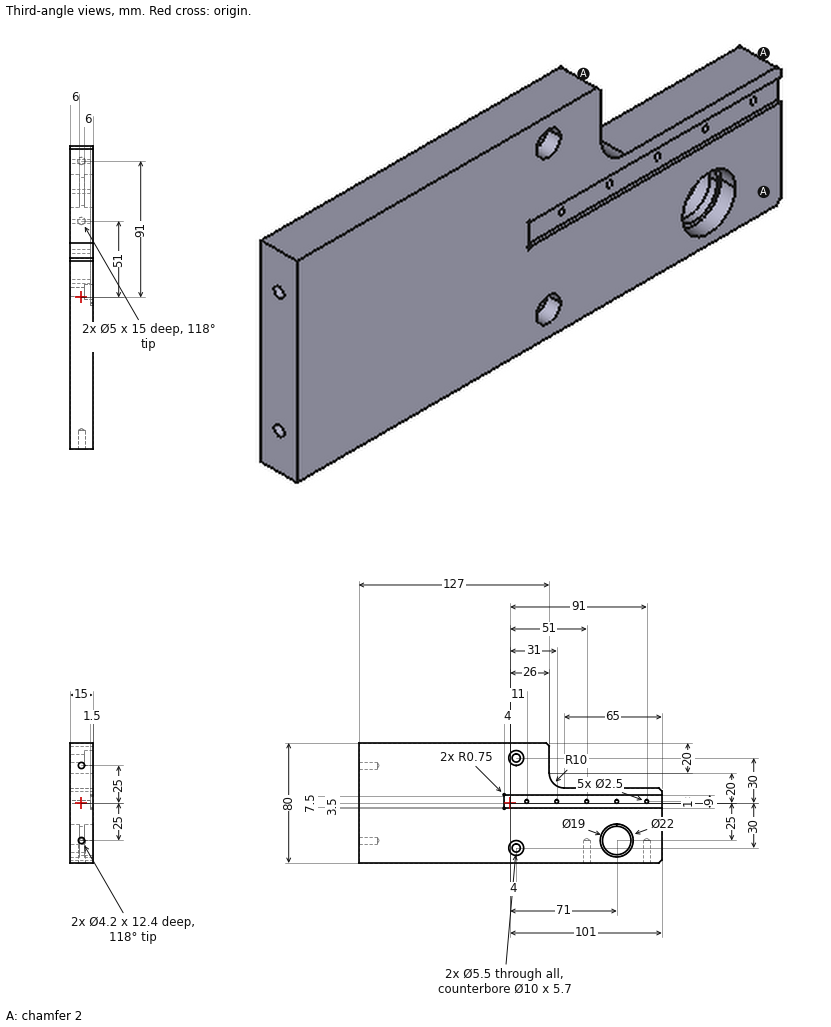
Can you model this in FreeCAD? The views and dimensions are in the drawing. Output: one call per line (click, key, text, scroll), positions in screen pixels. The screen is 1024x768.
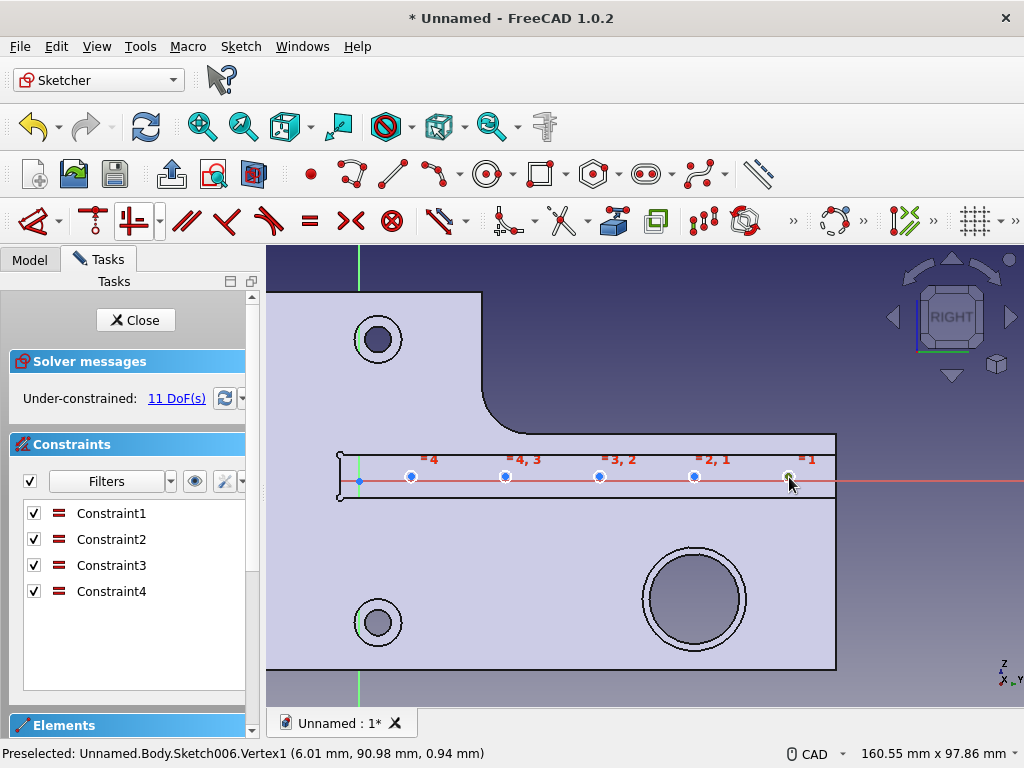
click(694, 477)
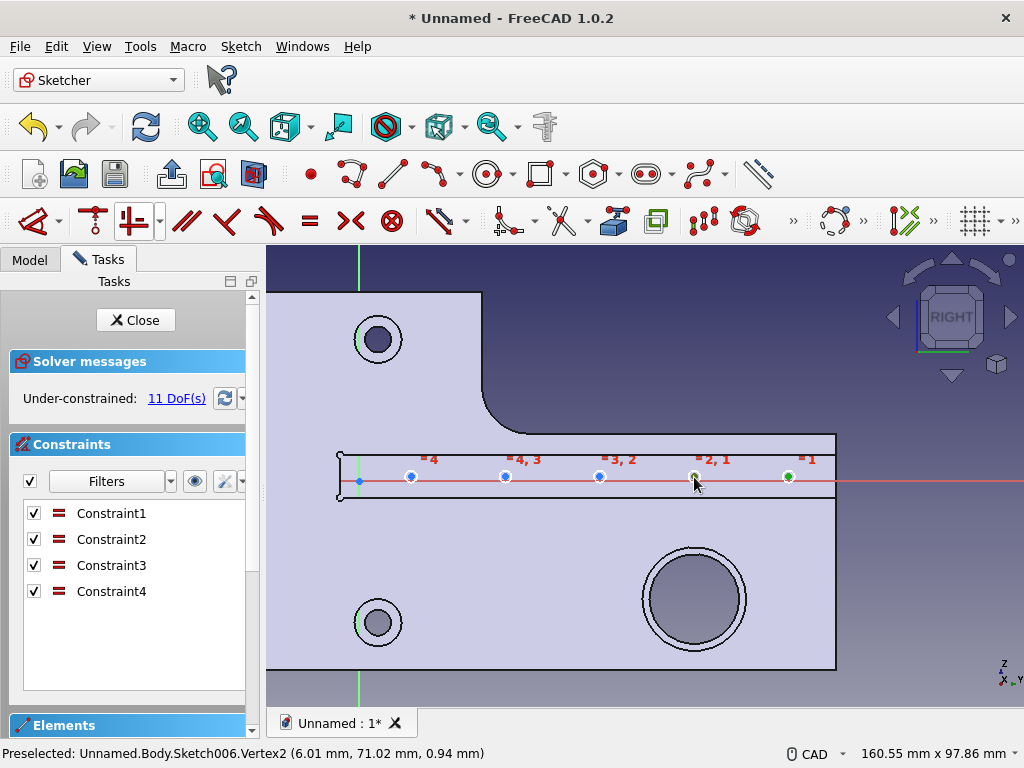
key(h)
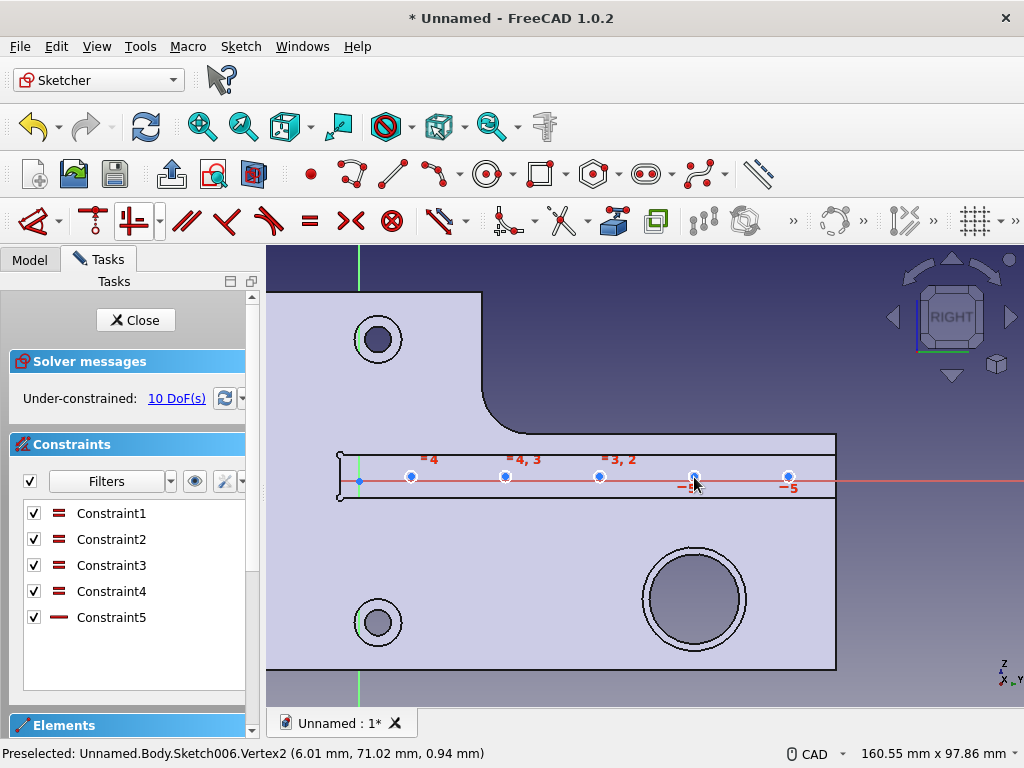
click(694, 477)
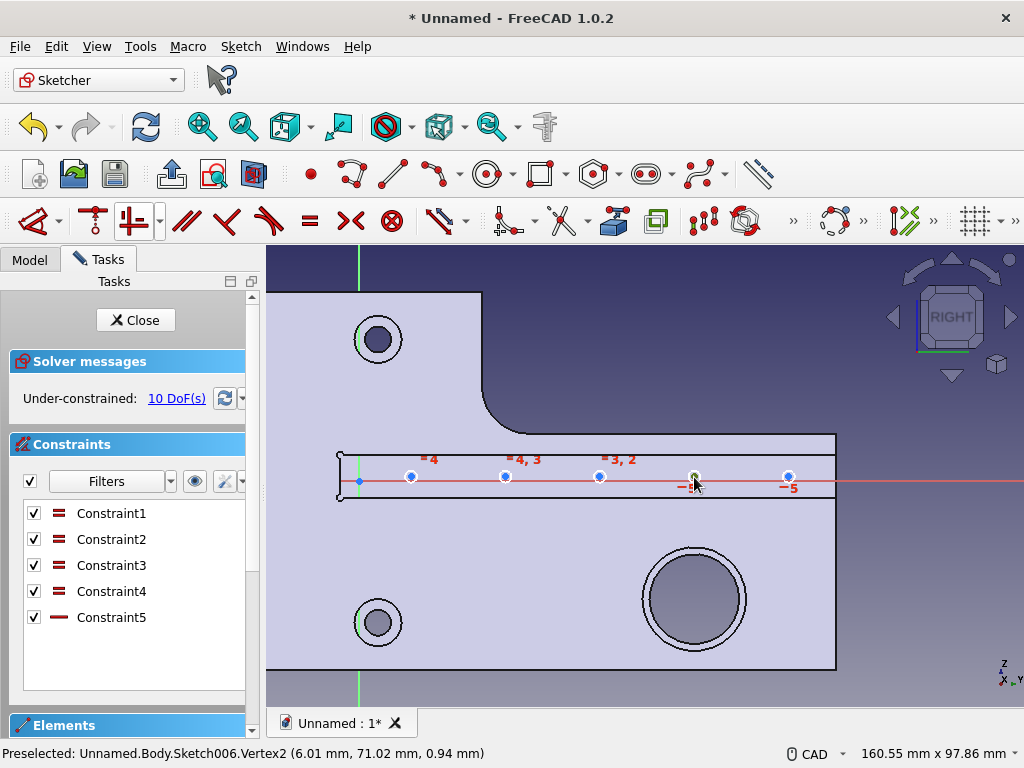
click(600, 477)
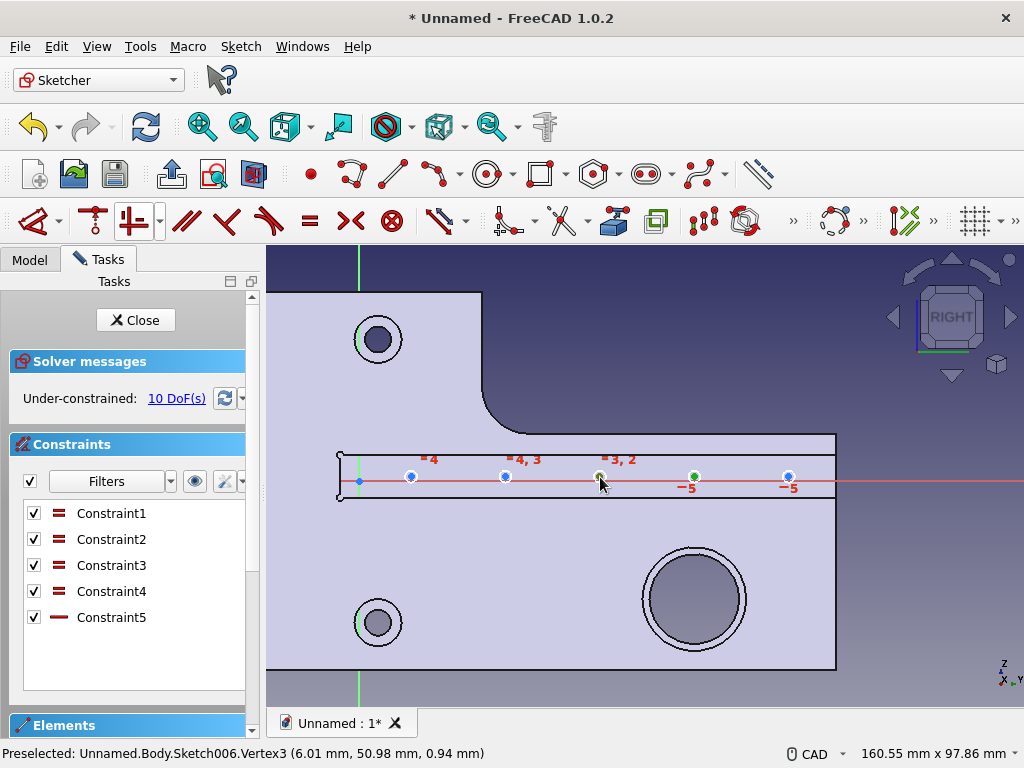
key(h)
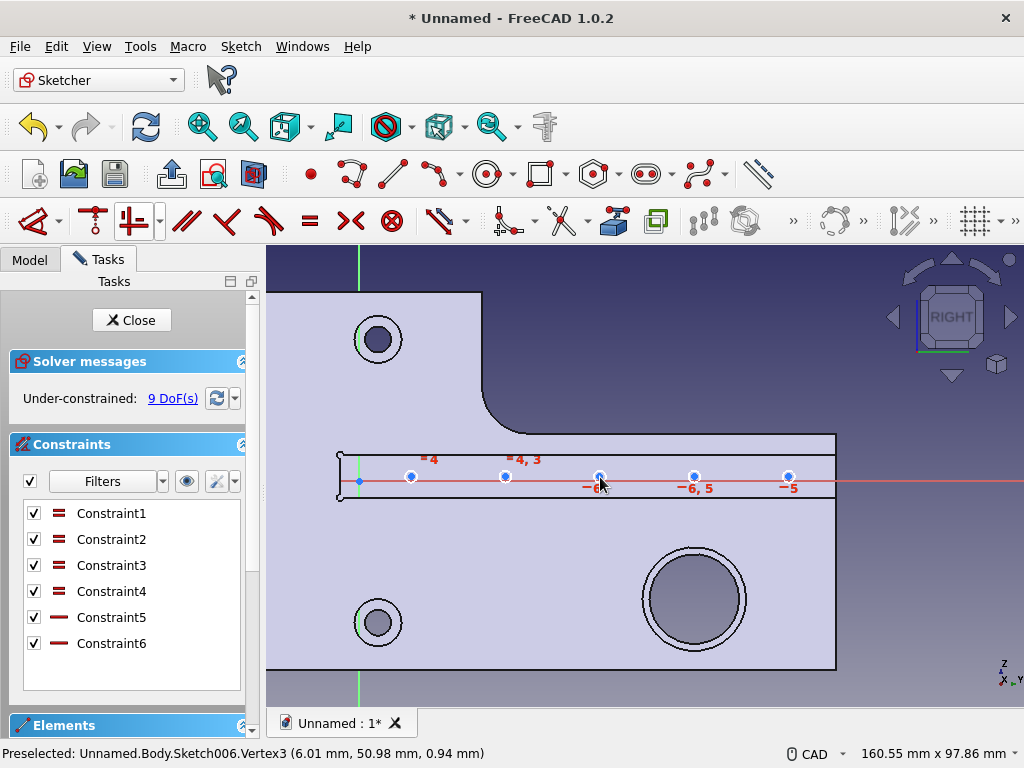
click(600, 477)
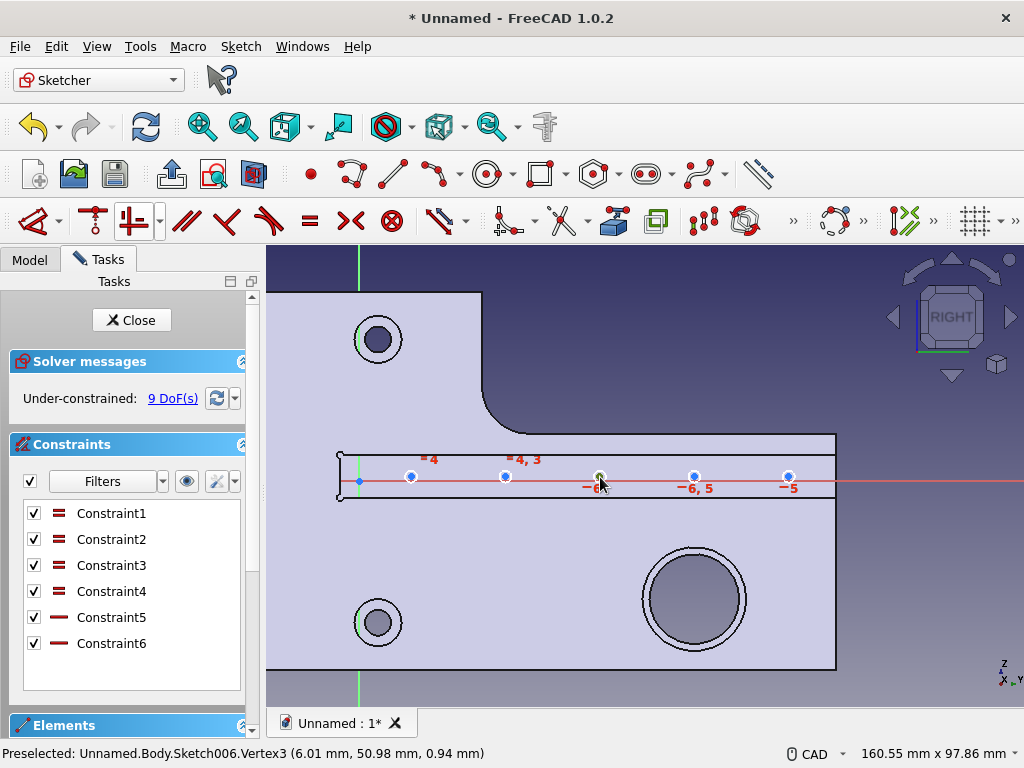
click(505, 477)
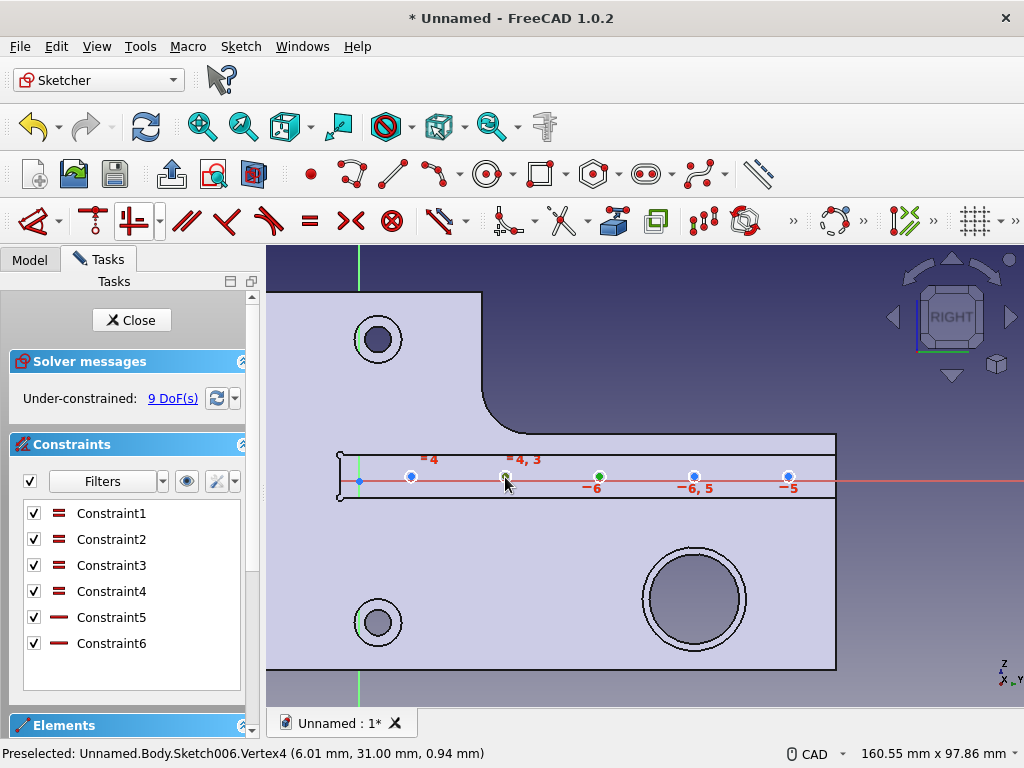
click(160, 222)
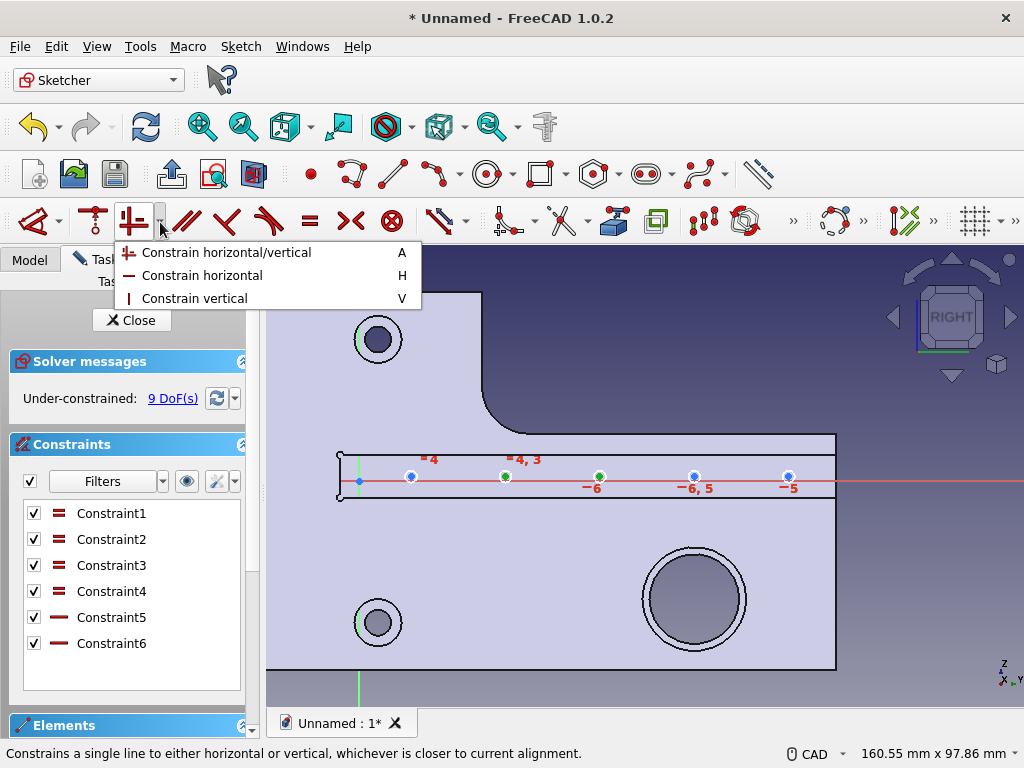
click(268, 276)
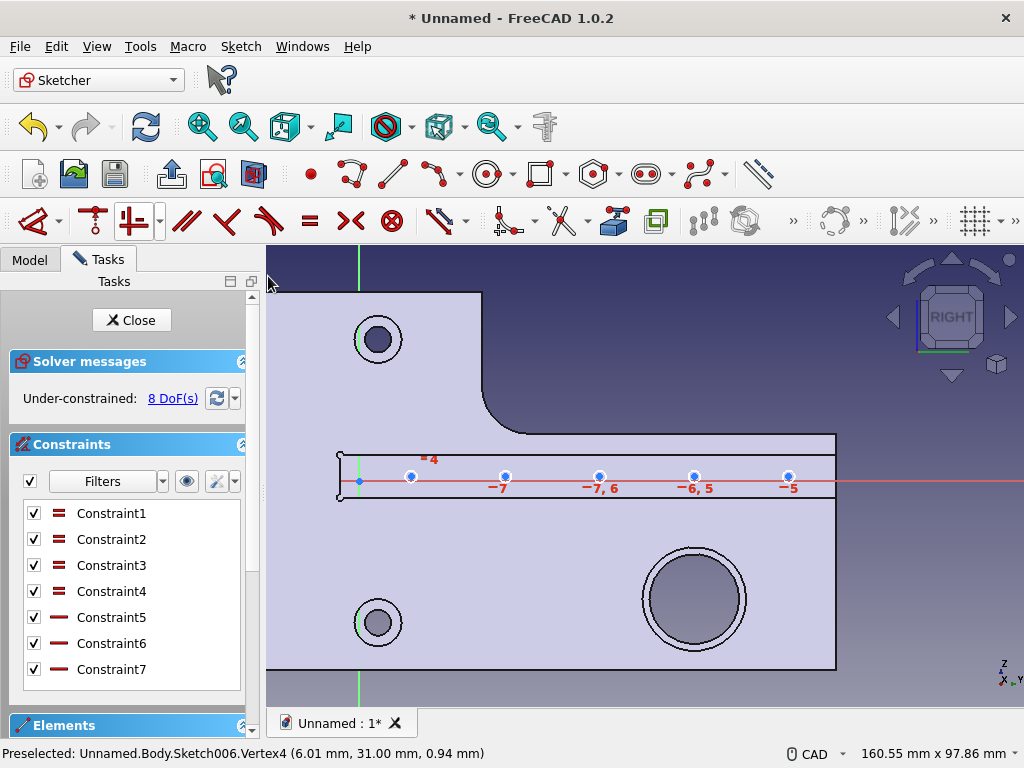
click(505, 477)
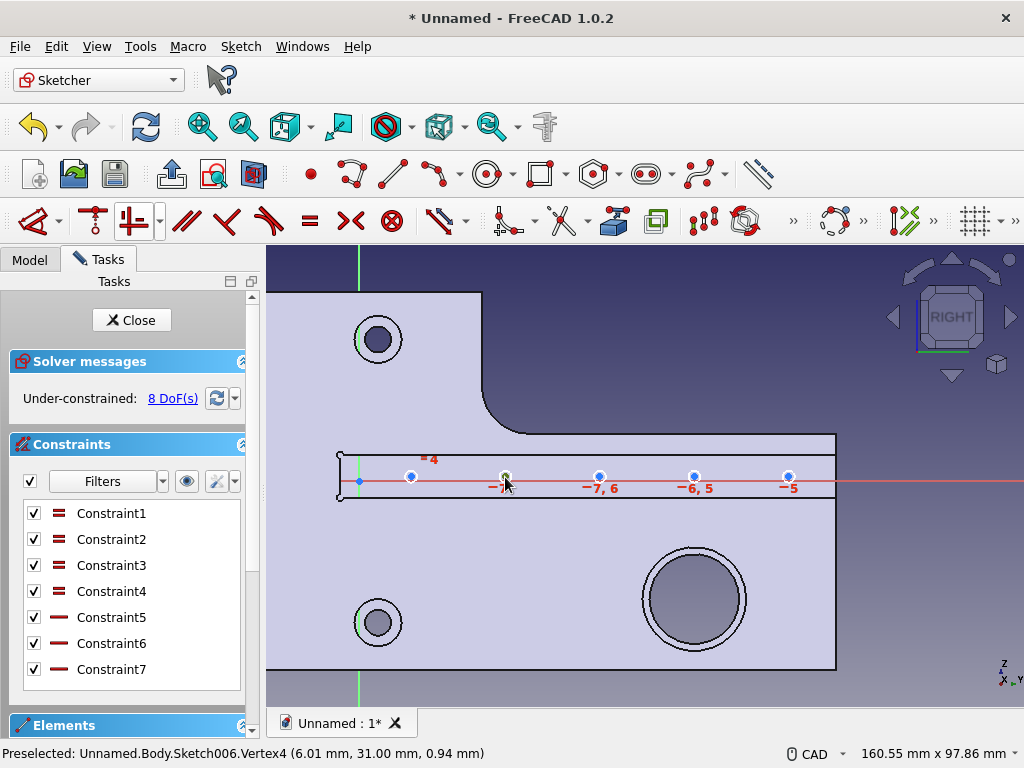
click(411, 477)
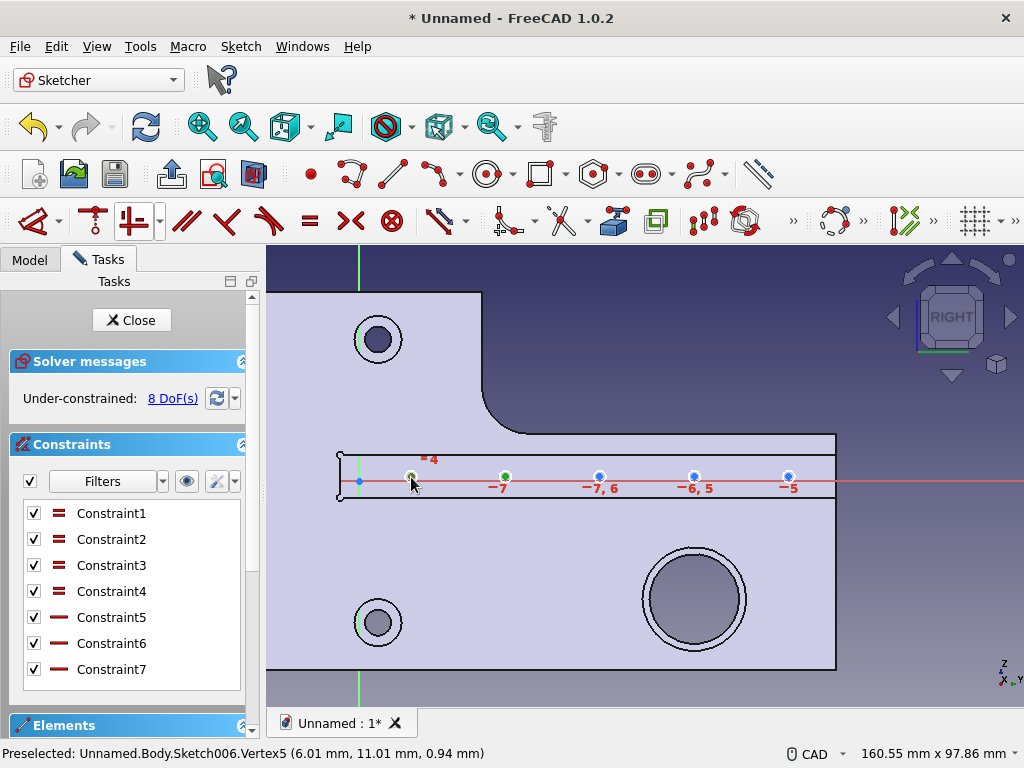
click(160, 222)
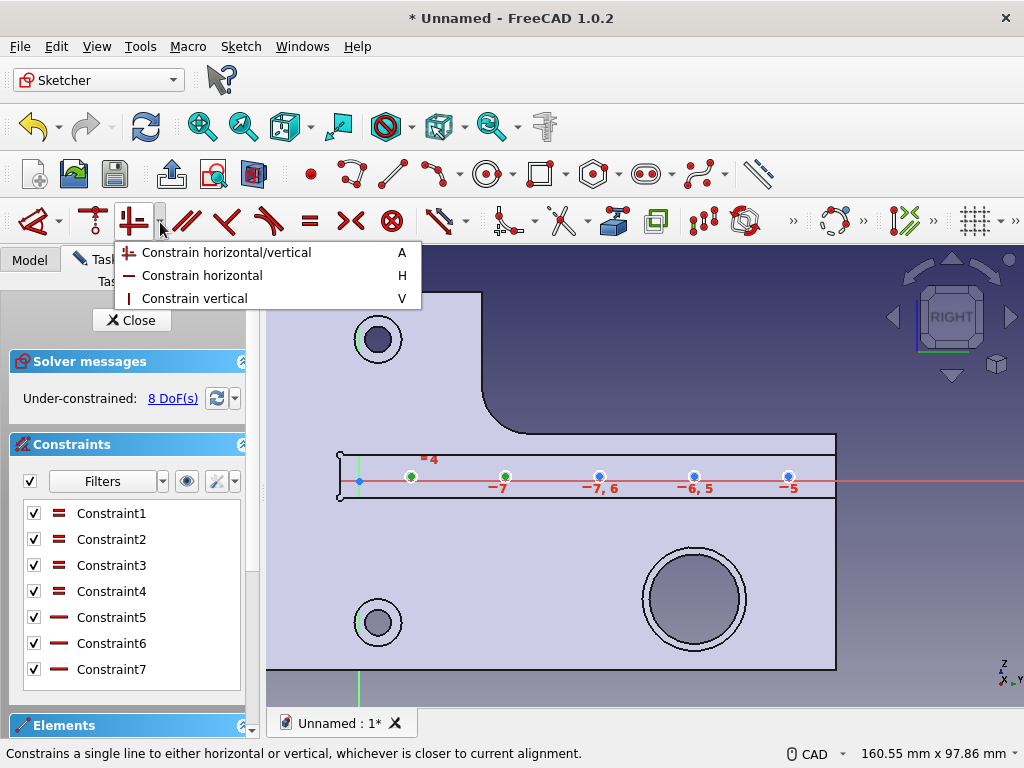
click(268, 276)